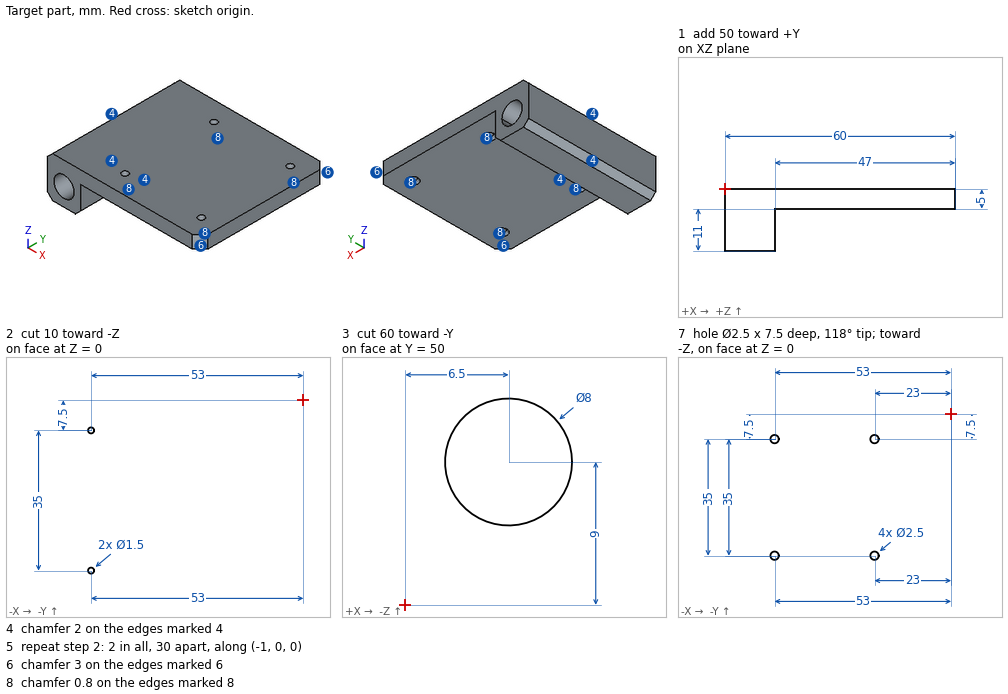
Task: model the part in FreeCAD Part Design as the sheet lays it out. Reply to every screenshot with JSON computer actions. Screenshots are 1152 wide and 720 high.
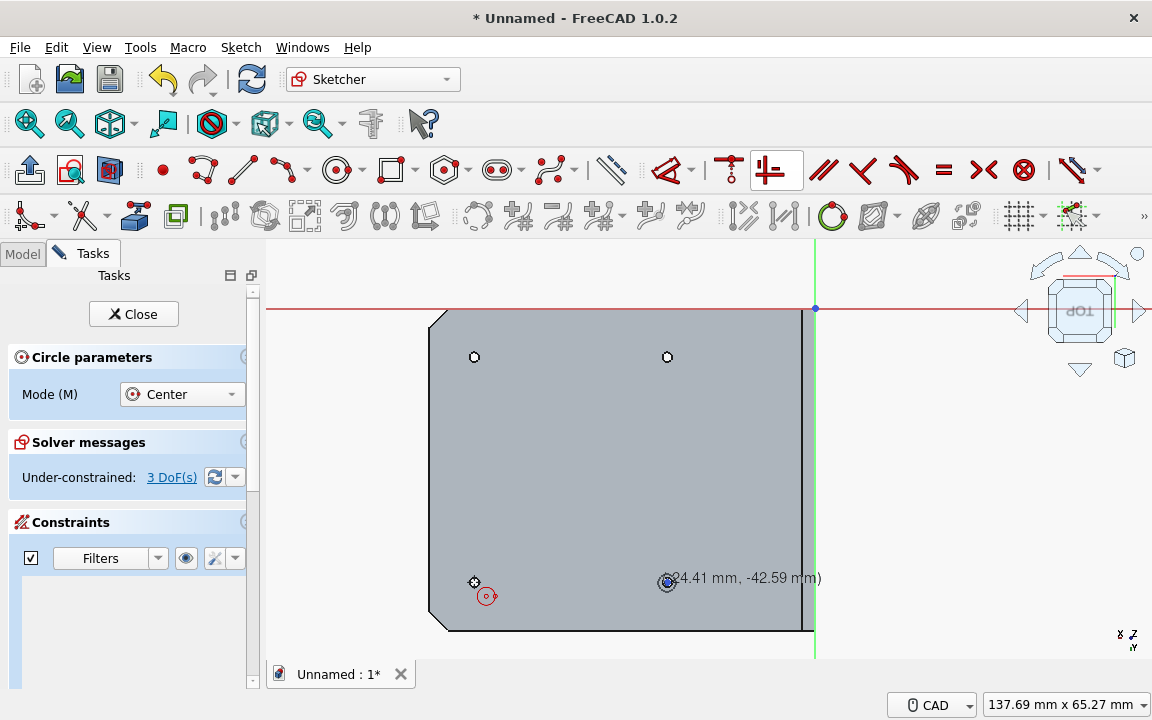
{"action": "left_click", "coordinate": [474, 582]}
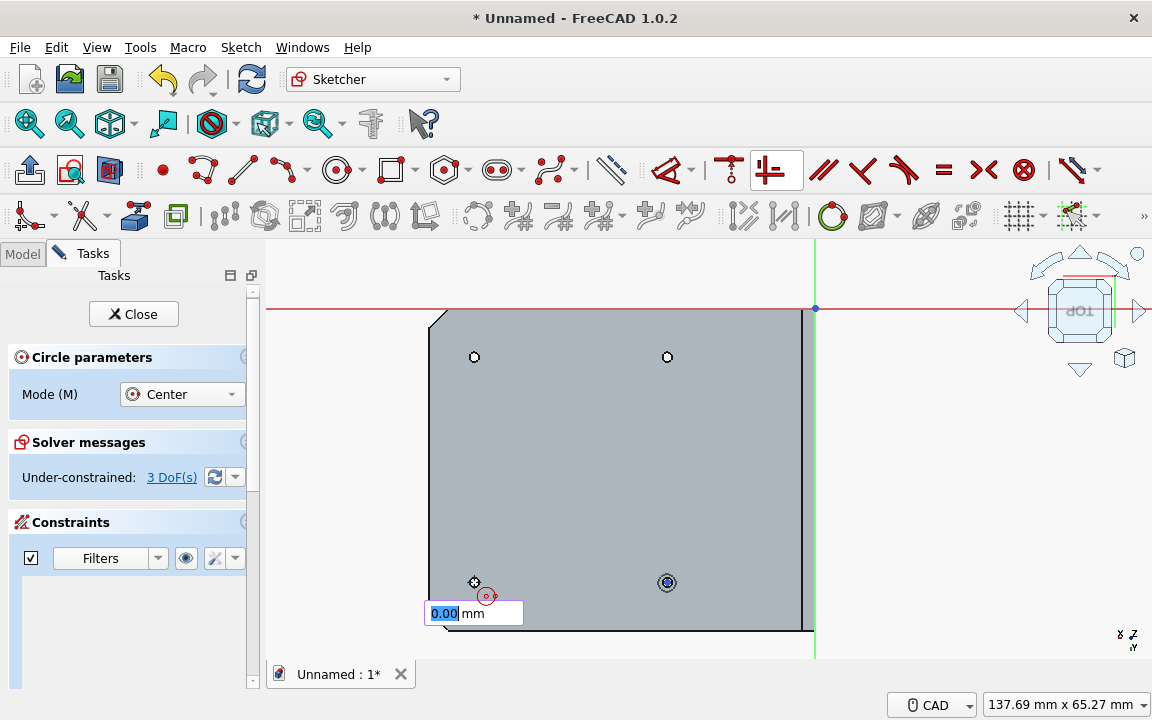
{"action": "scroll", "coordinate": [480, 577], "scroll_direction": "up", "scroll_amount": 4}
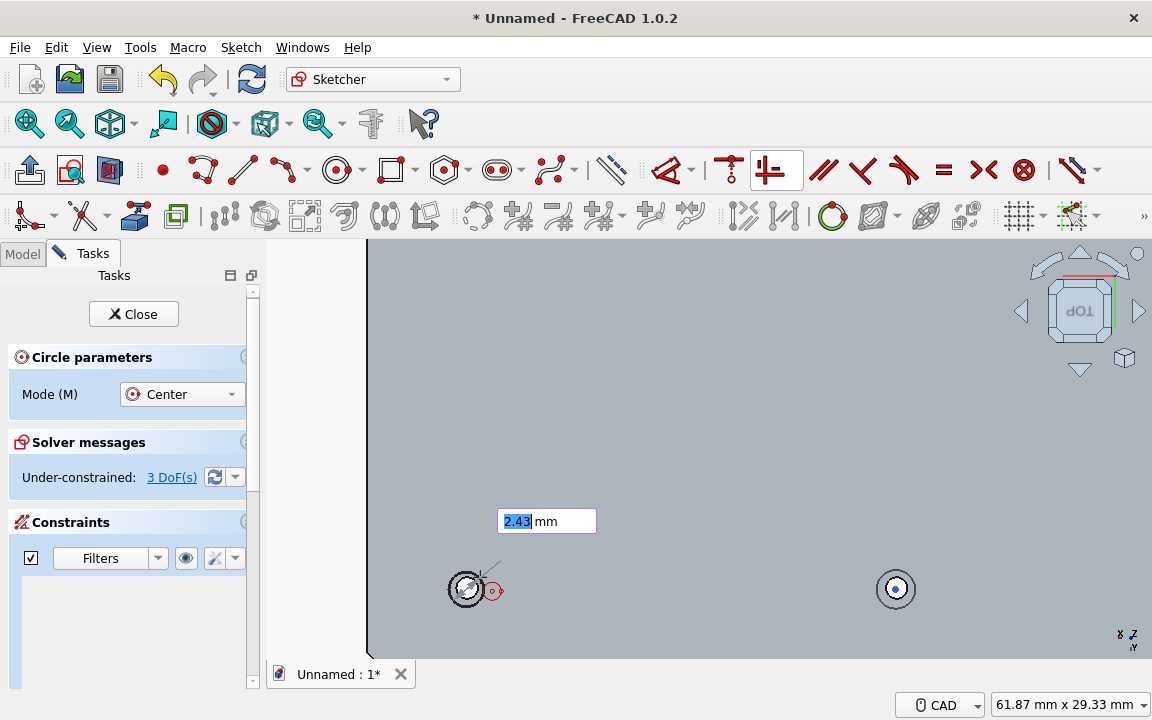
{"action": "left_click", "coordinate": [480, 575]}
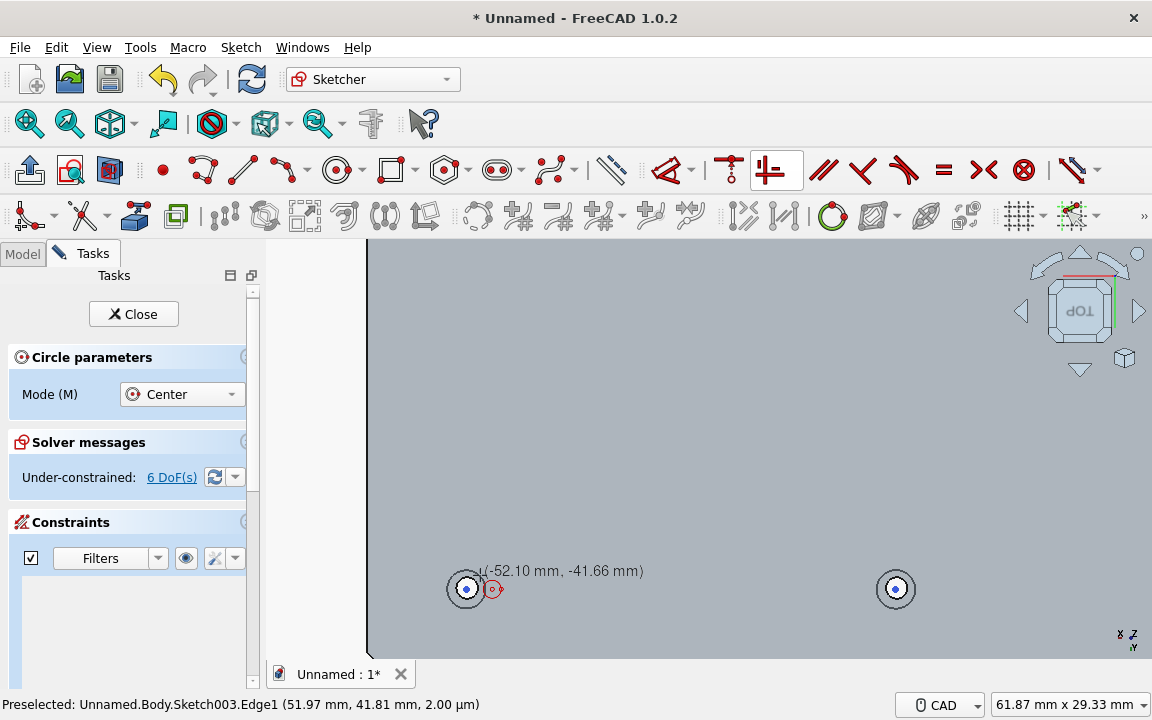
{"action": "scroll", "coordinate": [480, 577], "scroll_direction": "down", "scroll_amount": 4}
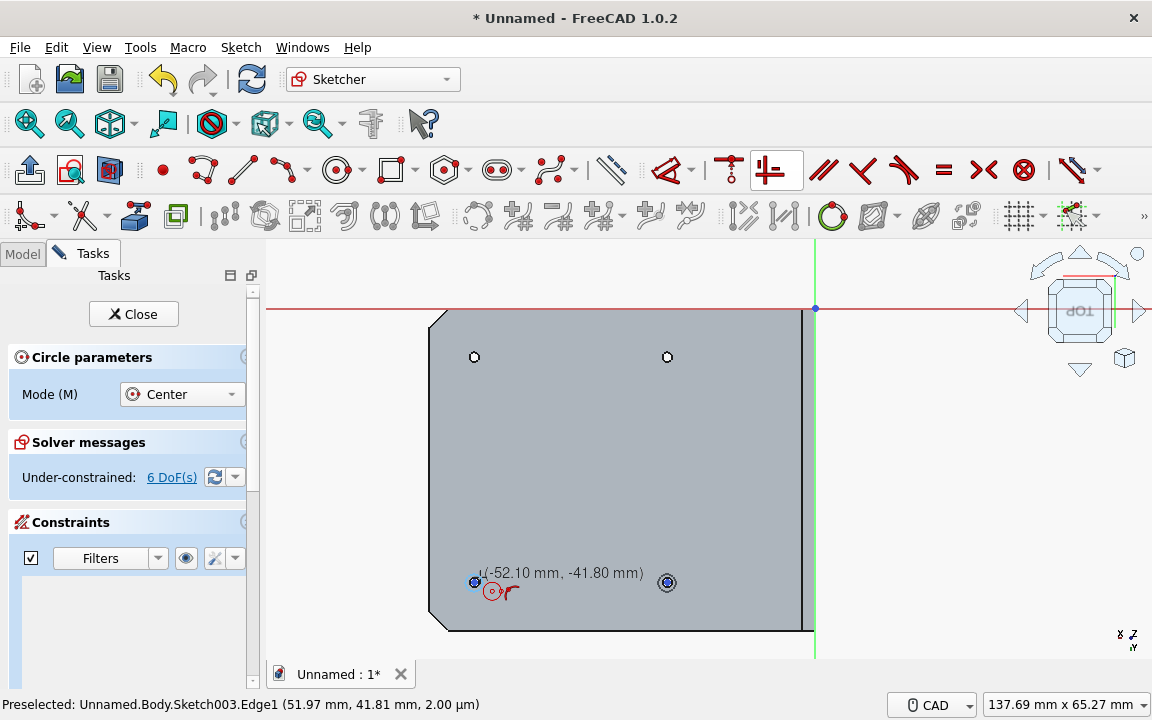
{"action": "scroll", "coordinate": [474, 357], "scroll_direction": "up", "scroll_amount": 6}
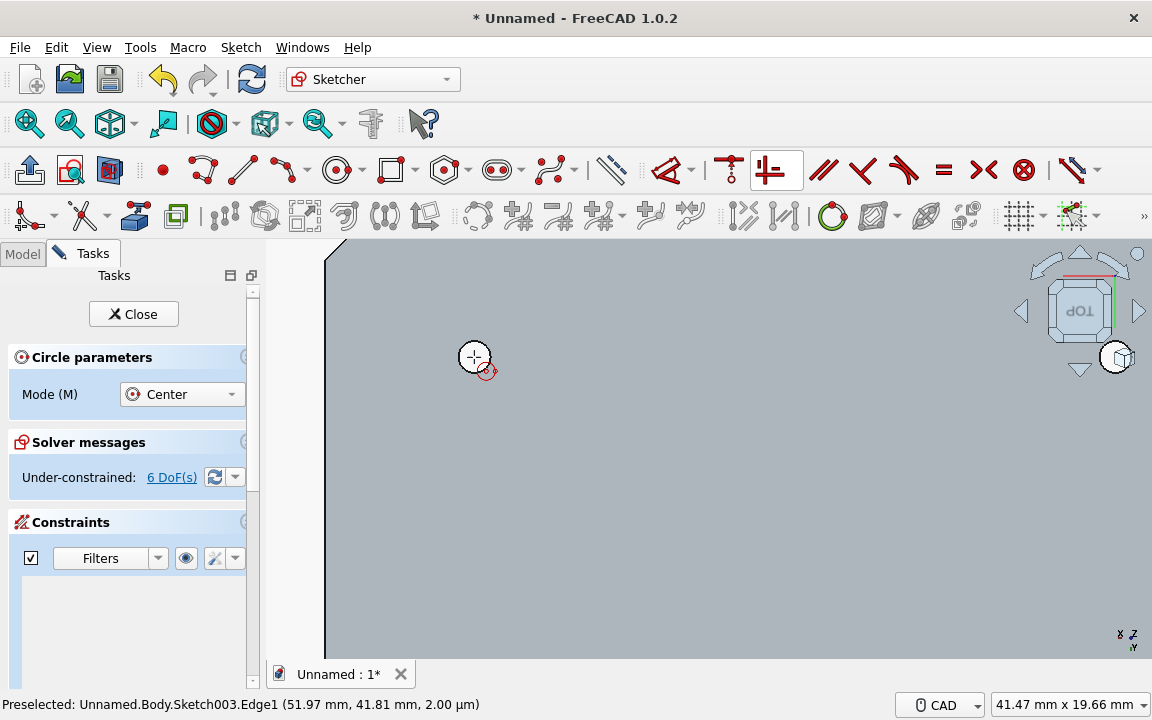
{"action": "scroll", "coordinate": [474, 356], "scroll_direction": "down", "scroll_amount": 6}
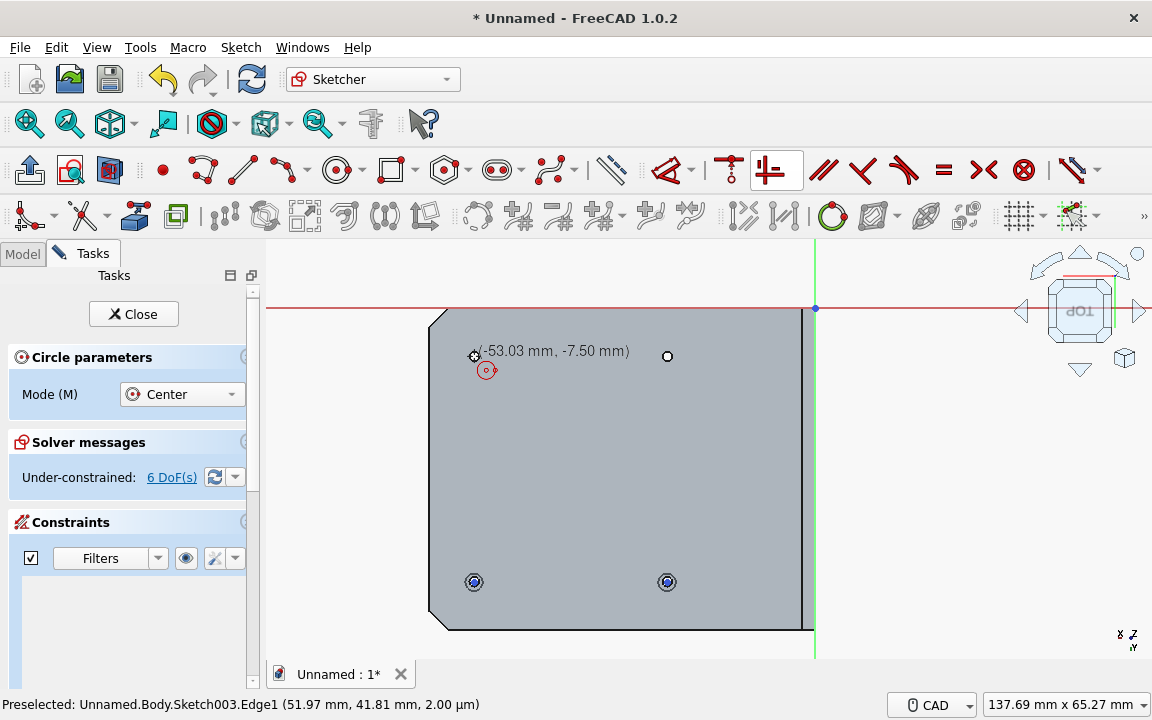
{"action": "left_click", "coordinate": [474, 356]}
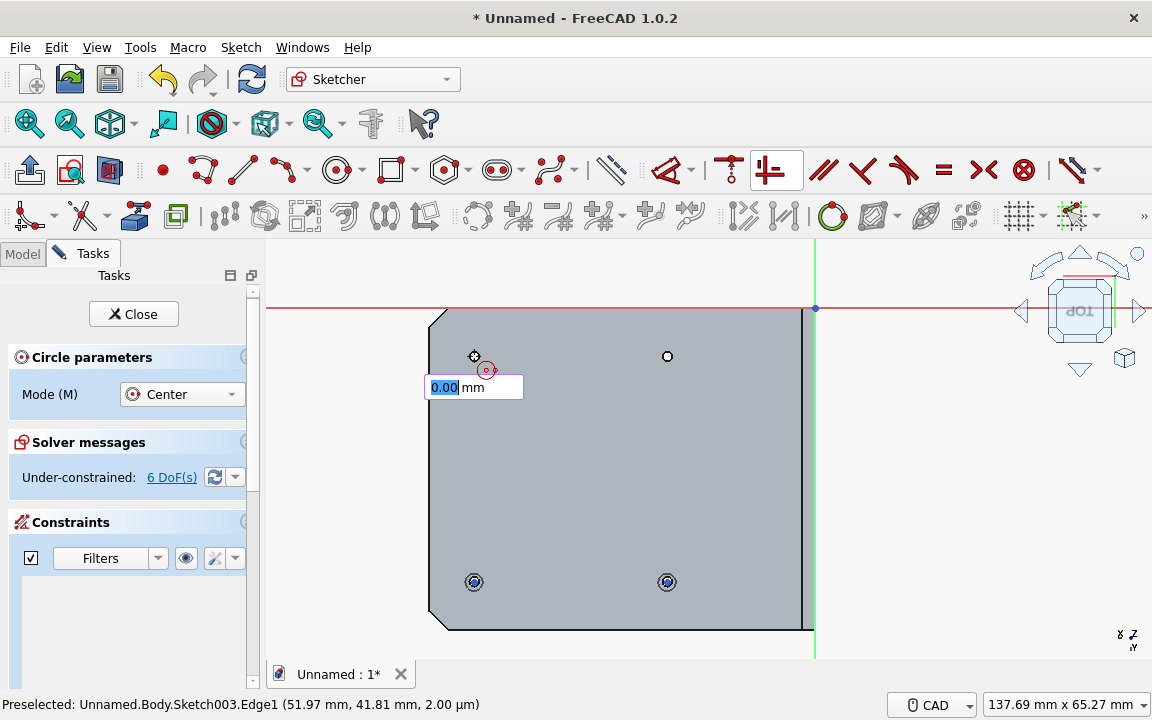
{"action": "scroll", "coordinate": [480, 351], "scroll_direction": "up", "scroll_amount": 4}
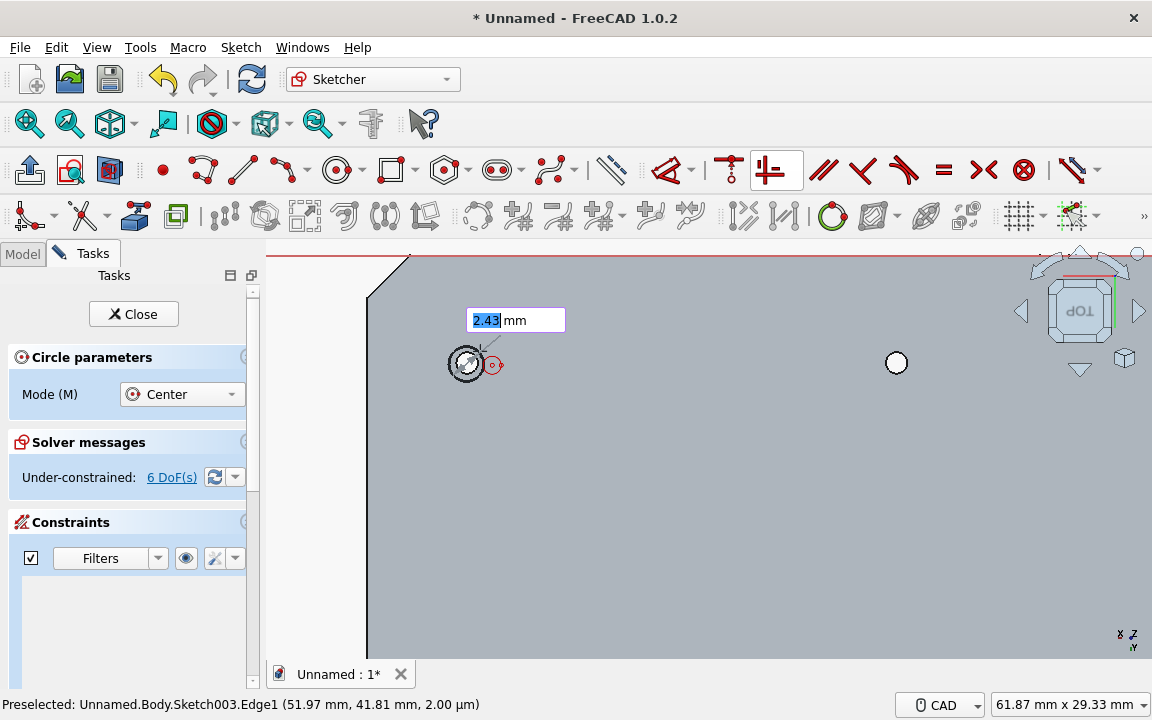
{"action": "left_click", "coordinate": [480, 350]}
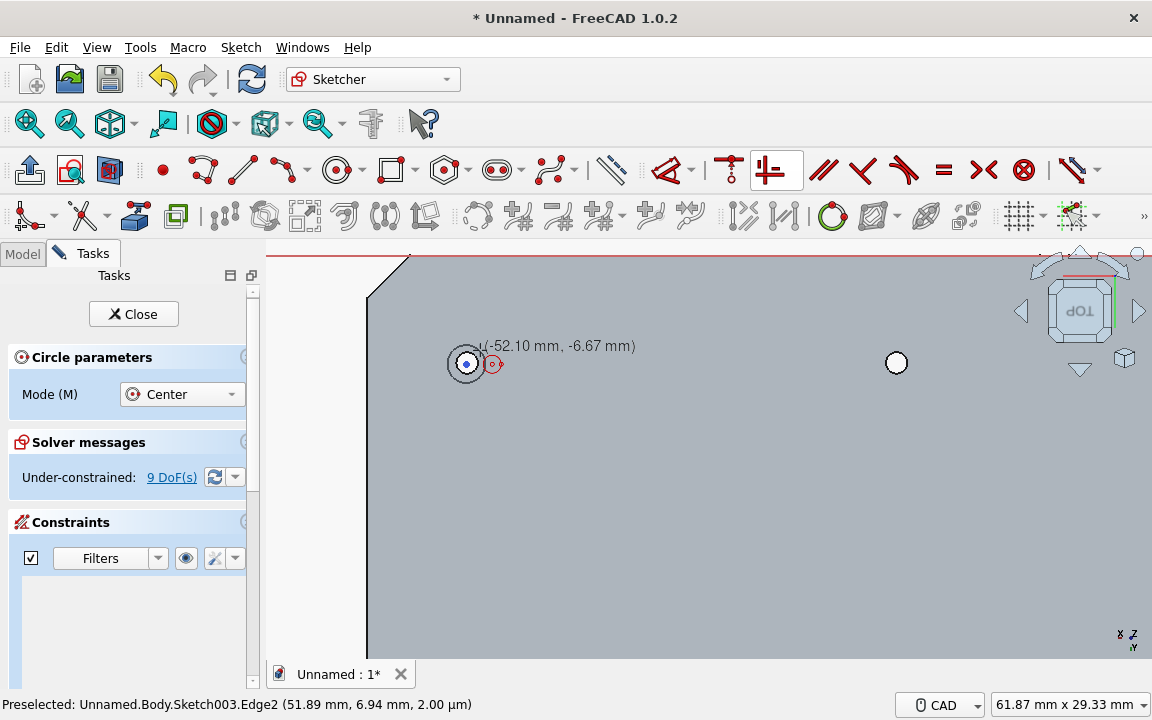
{"action": "scroll", "coordinate": [897, 363], "scroll_direction": "up", "scroll_amount": 2}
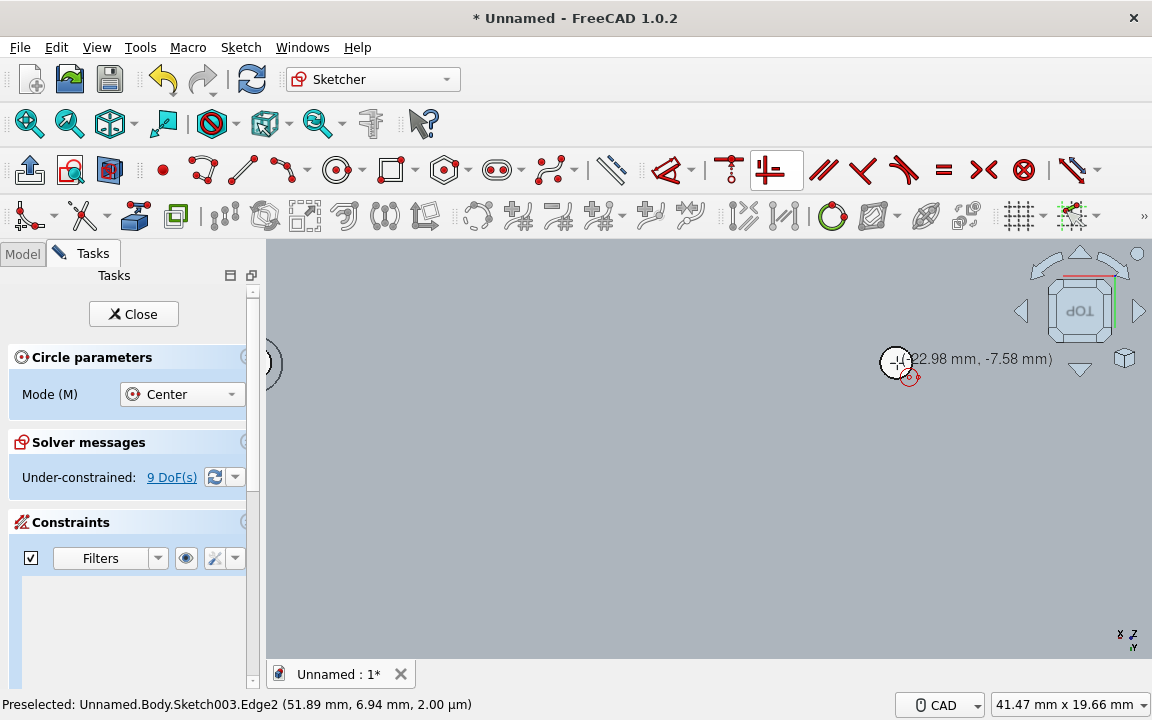
{"action": "scroll", "coordinate": [568, 354], "scroll_direction": "down", "scroll_amount": 6}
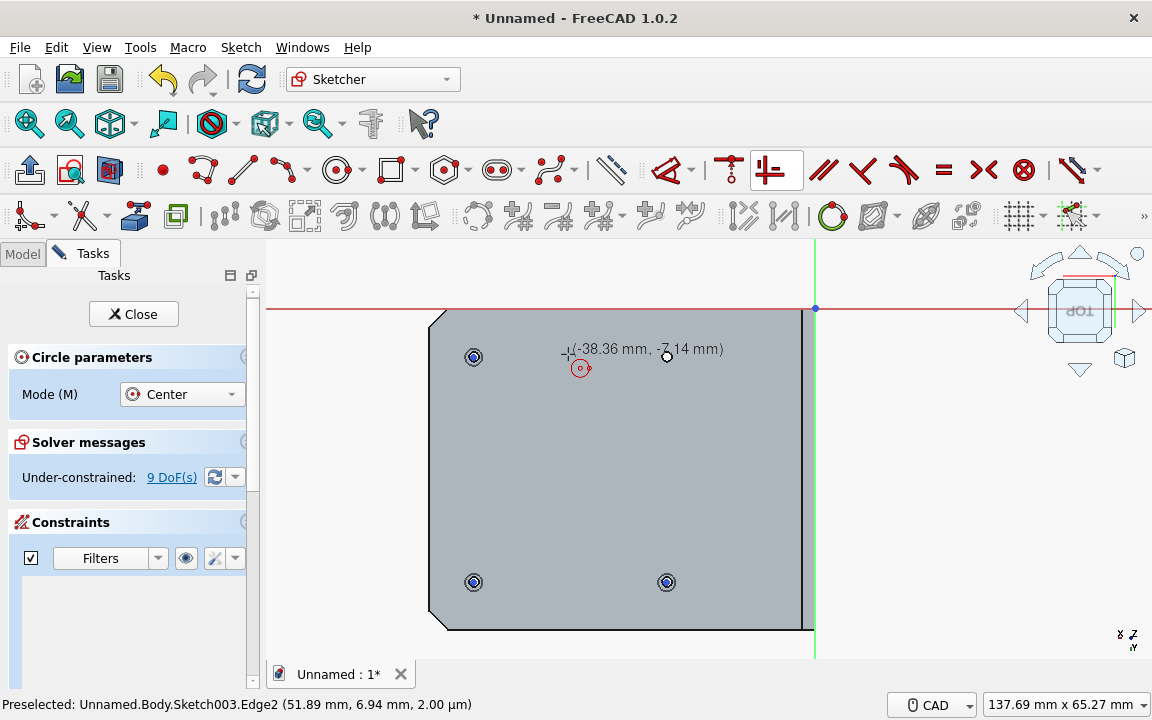
{"action": "left_click", "coordinate": [667, 357]}